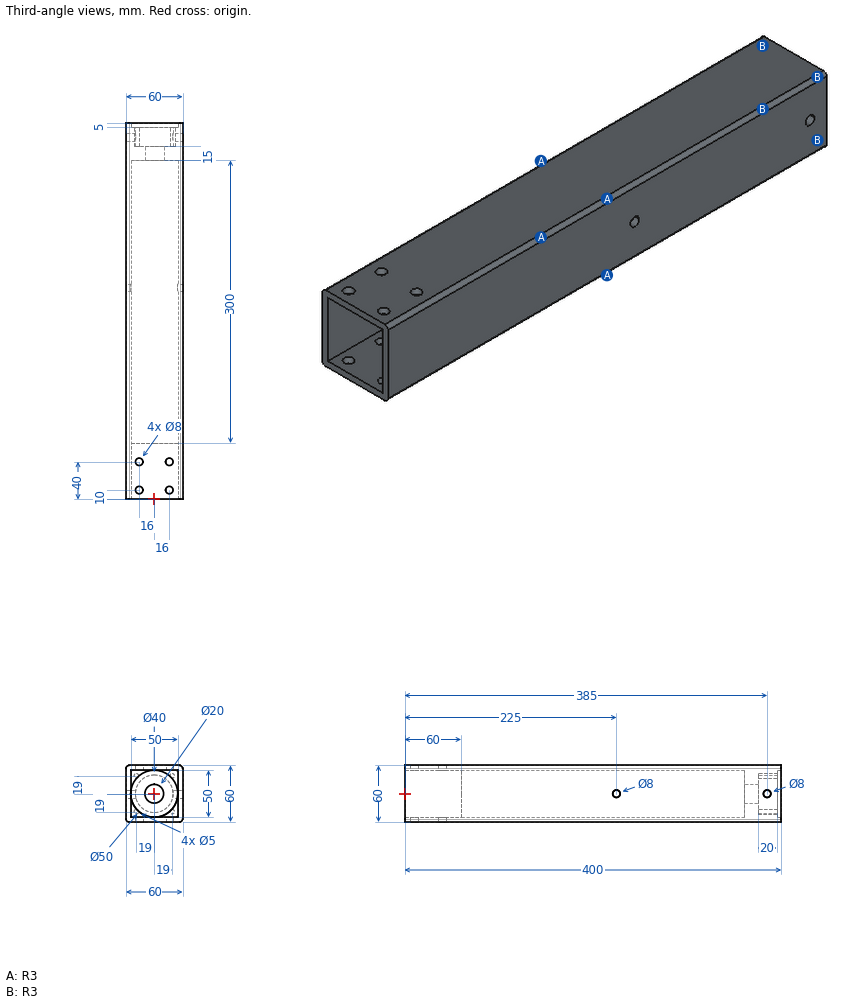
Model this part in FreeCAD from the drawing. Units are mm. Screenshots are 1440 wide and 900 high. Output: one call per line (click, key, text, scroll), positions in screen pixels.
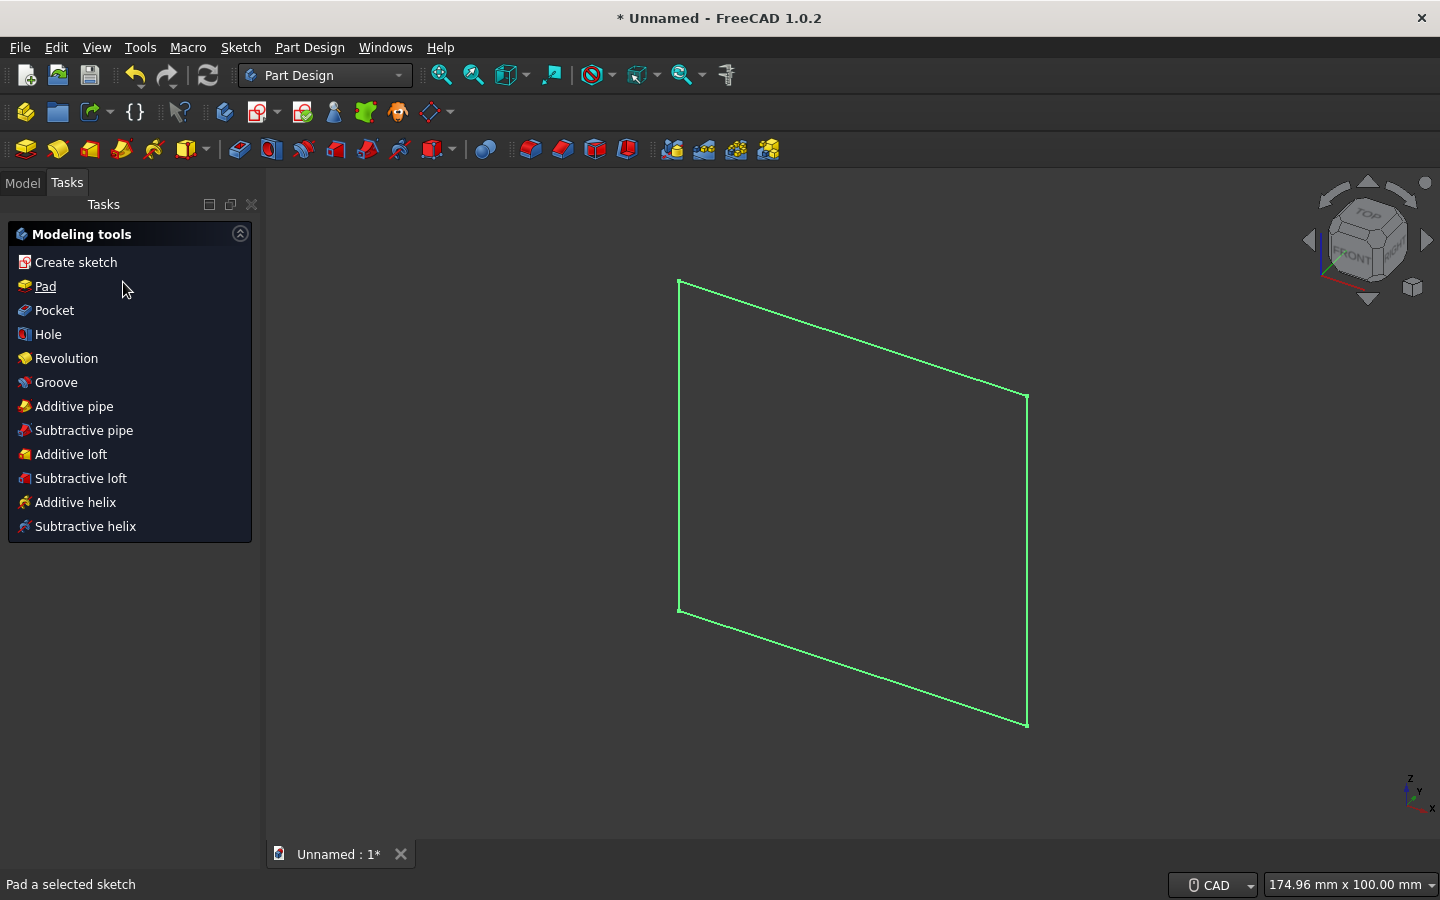
click(26, 150)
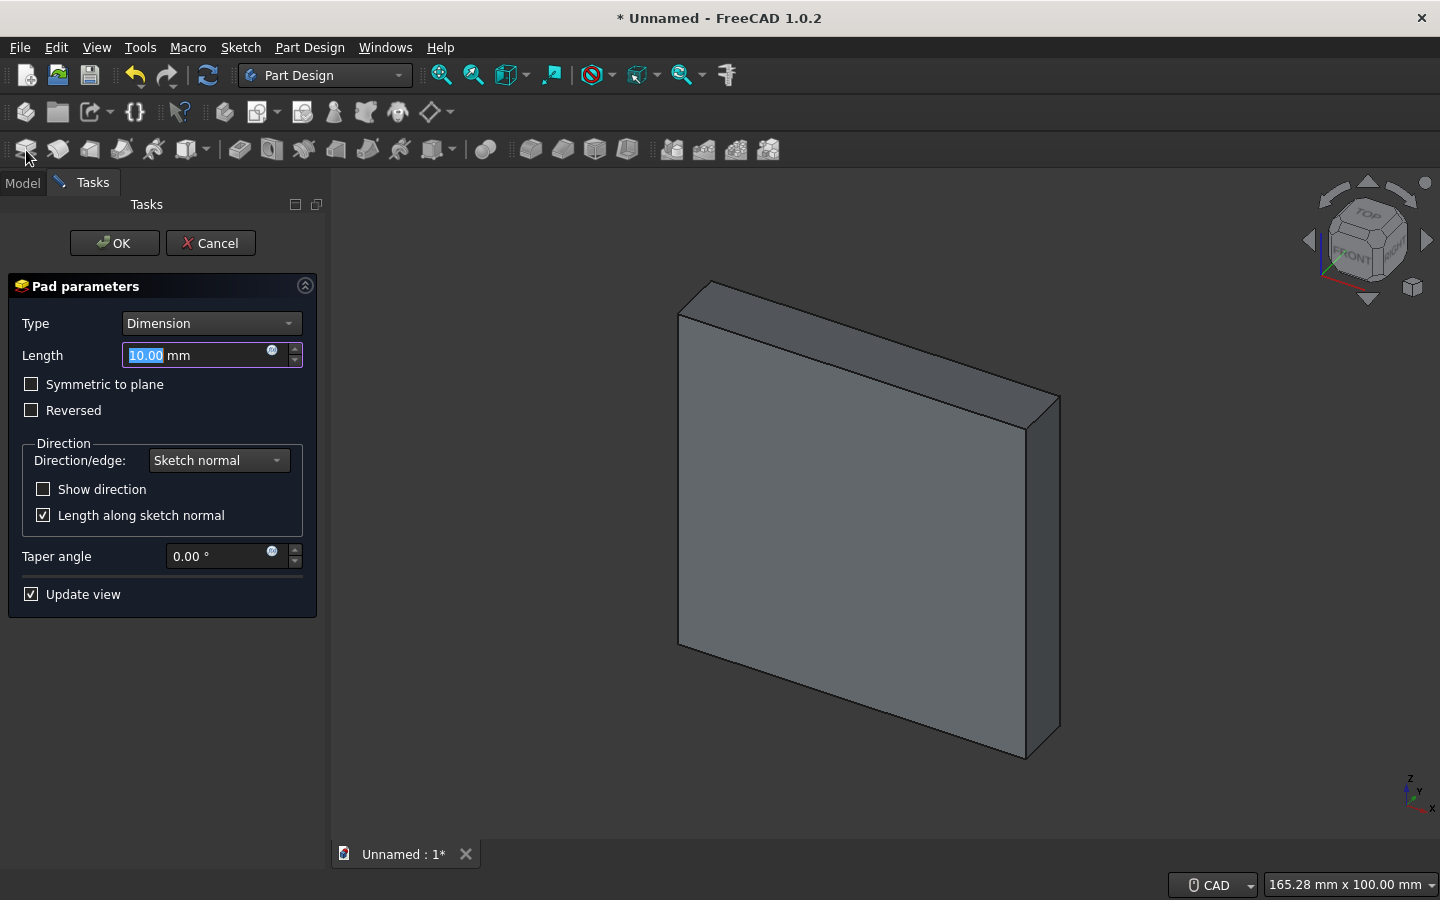
text(400)
key(Tab)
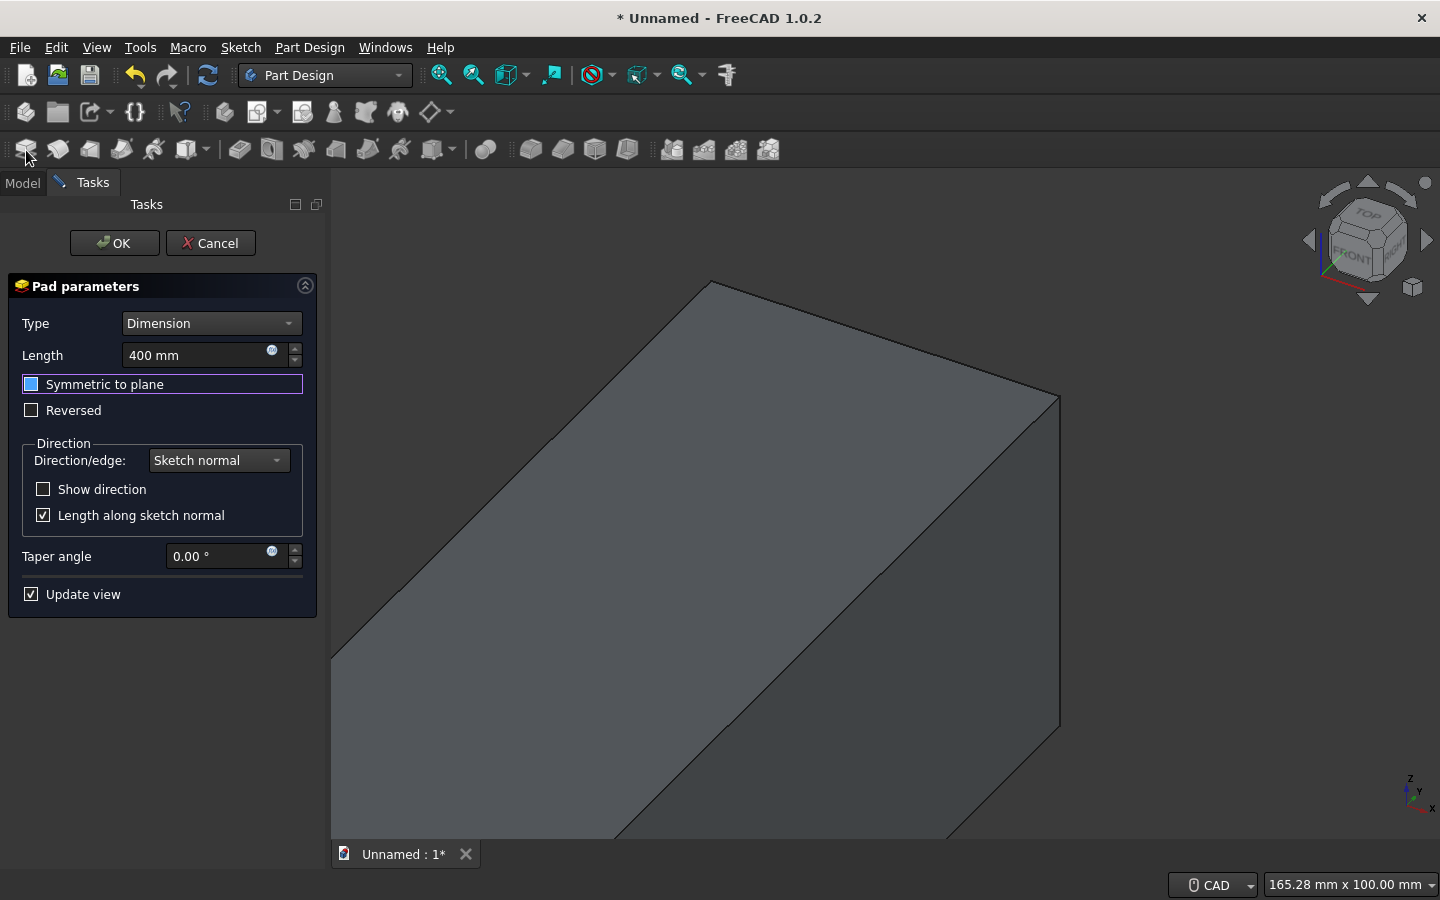
click(30, 410)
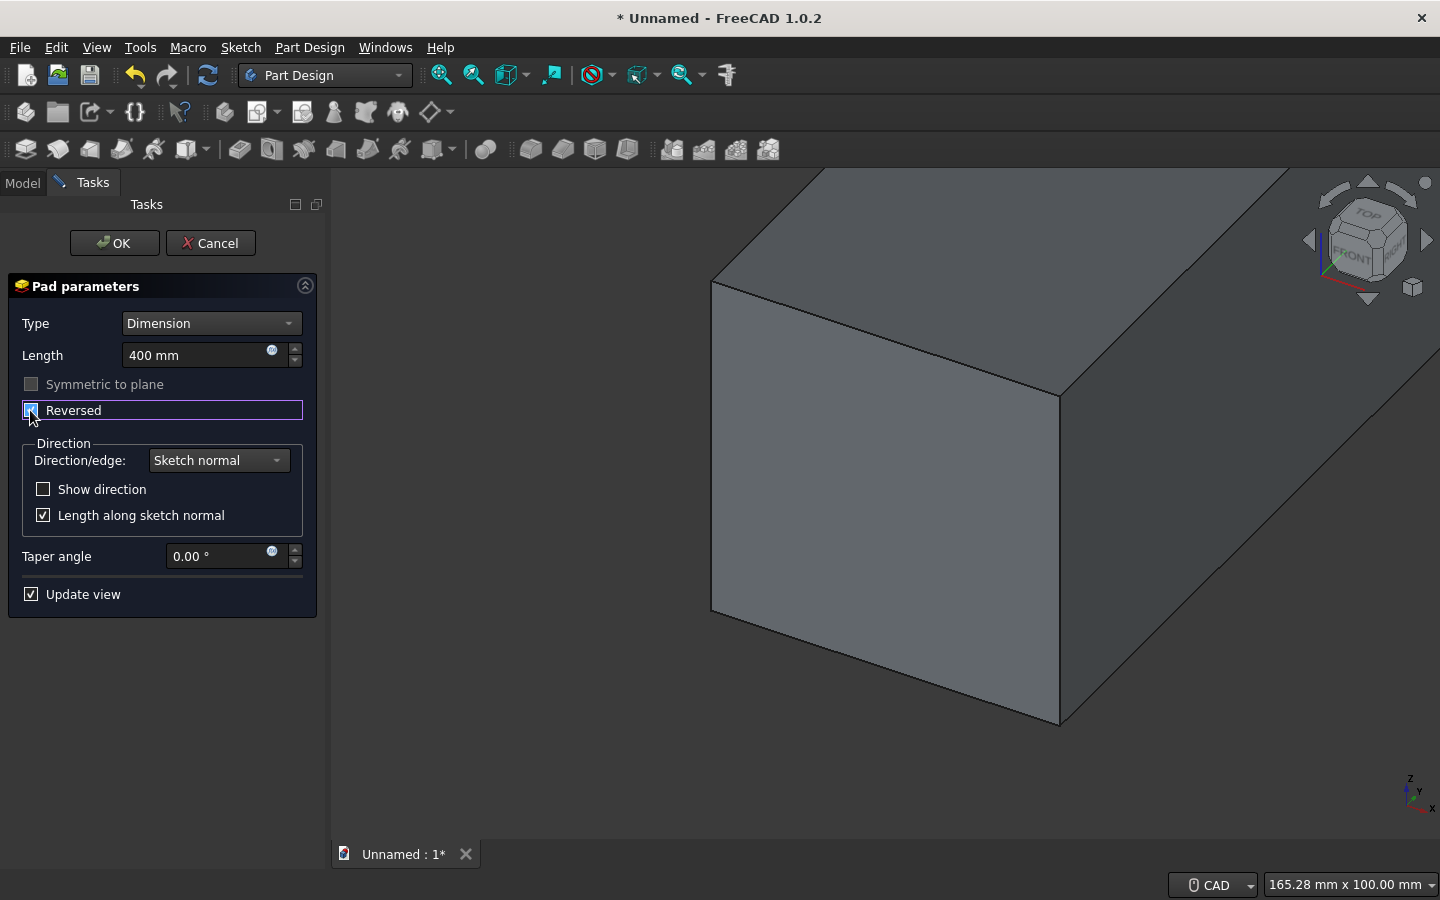
click(115, 243)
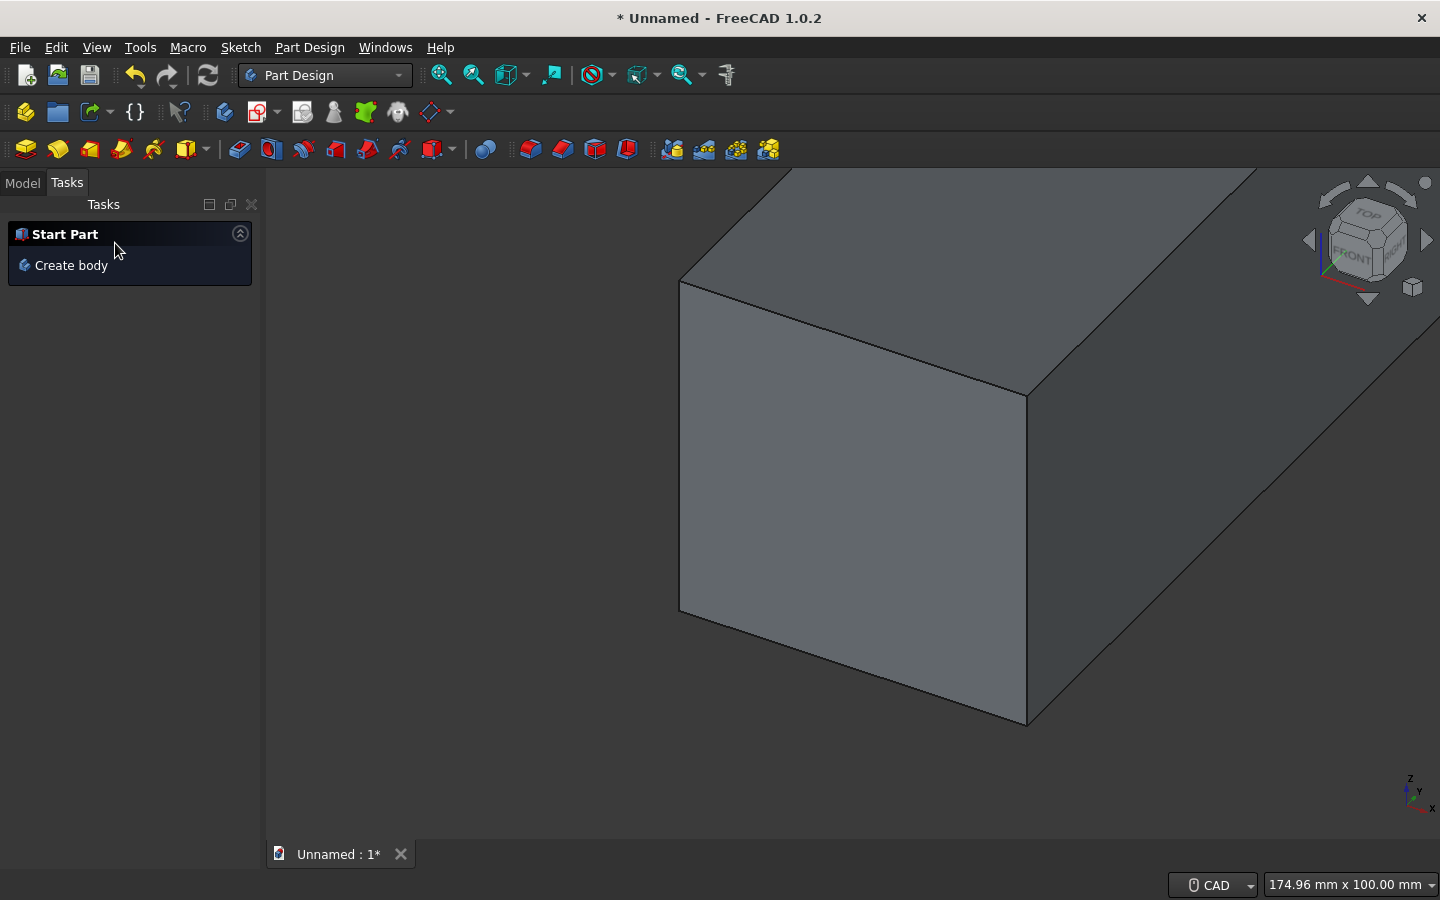
click(442, 76)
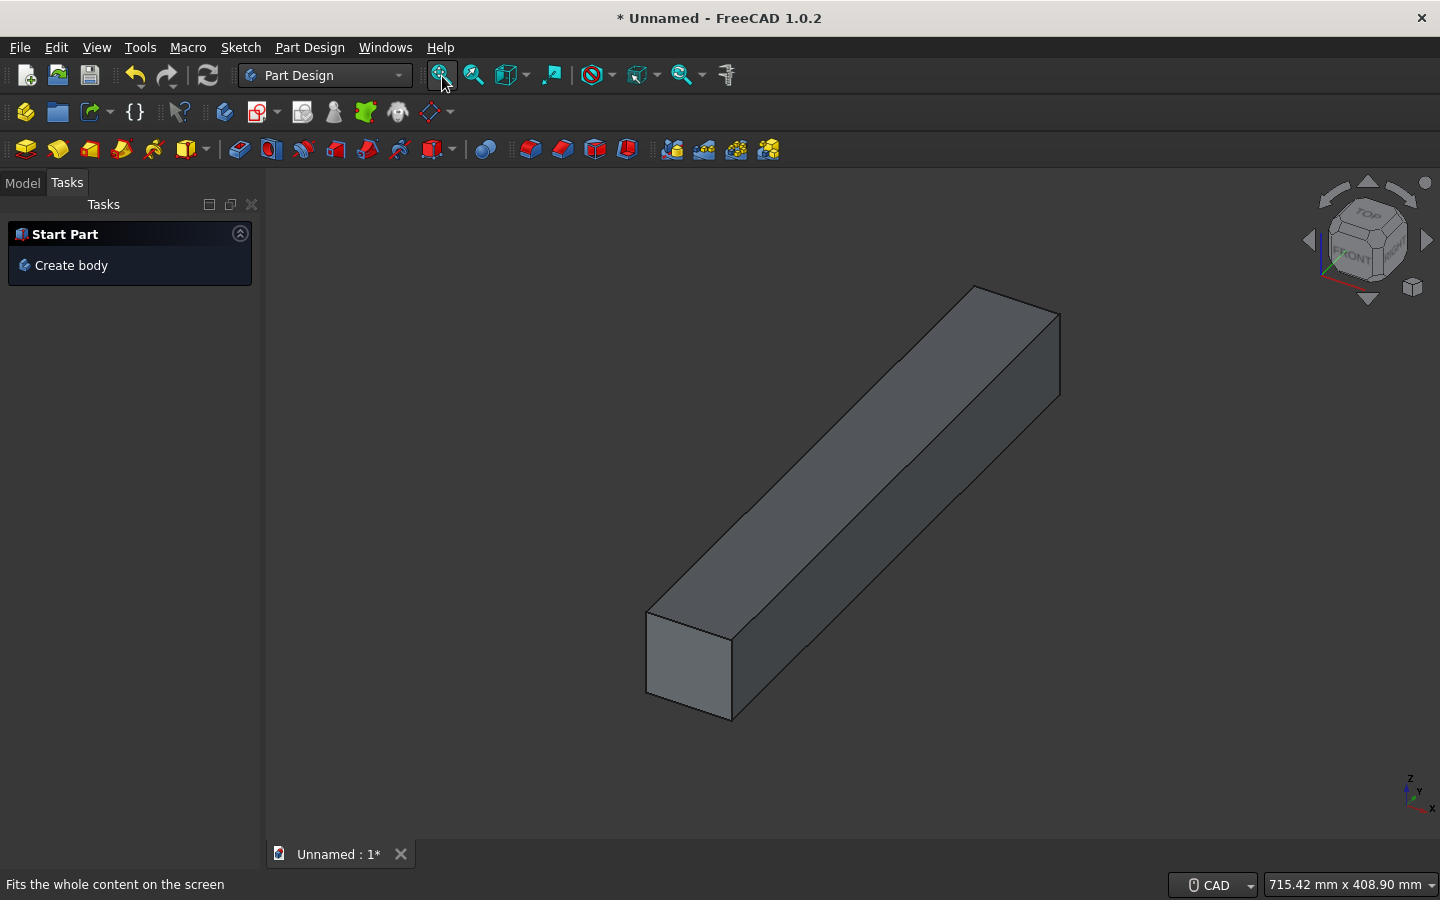
key(4)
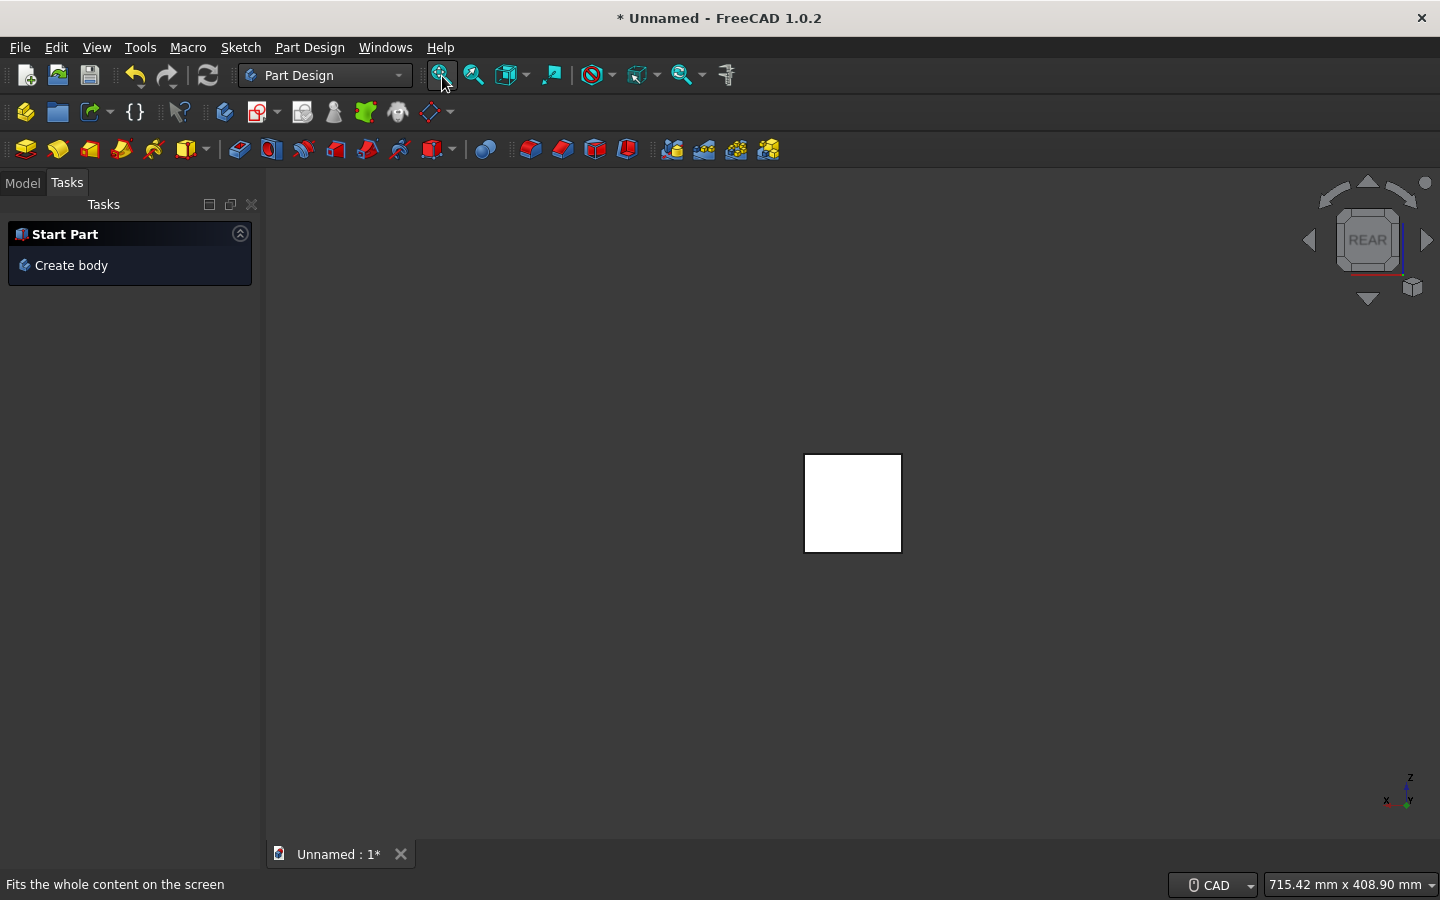
click(442, 76)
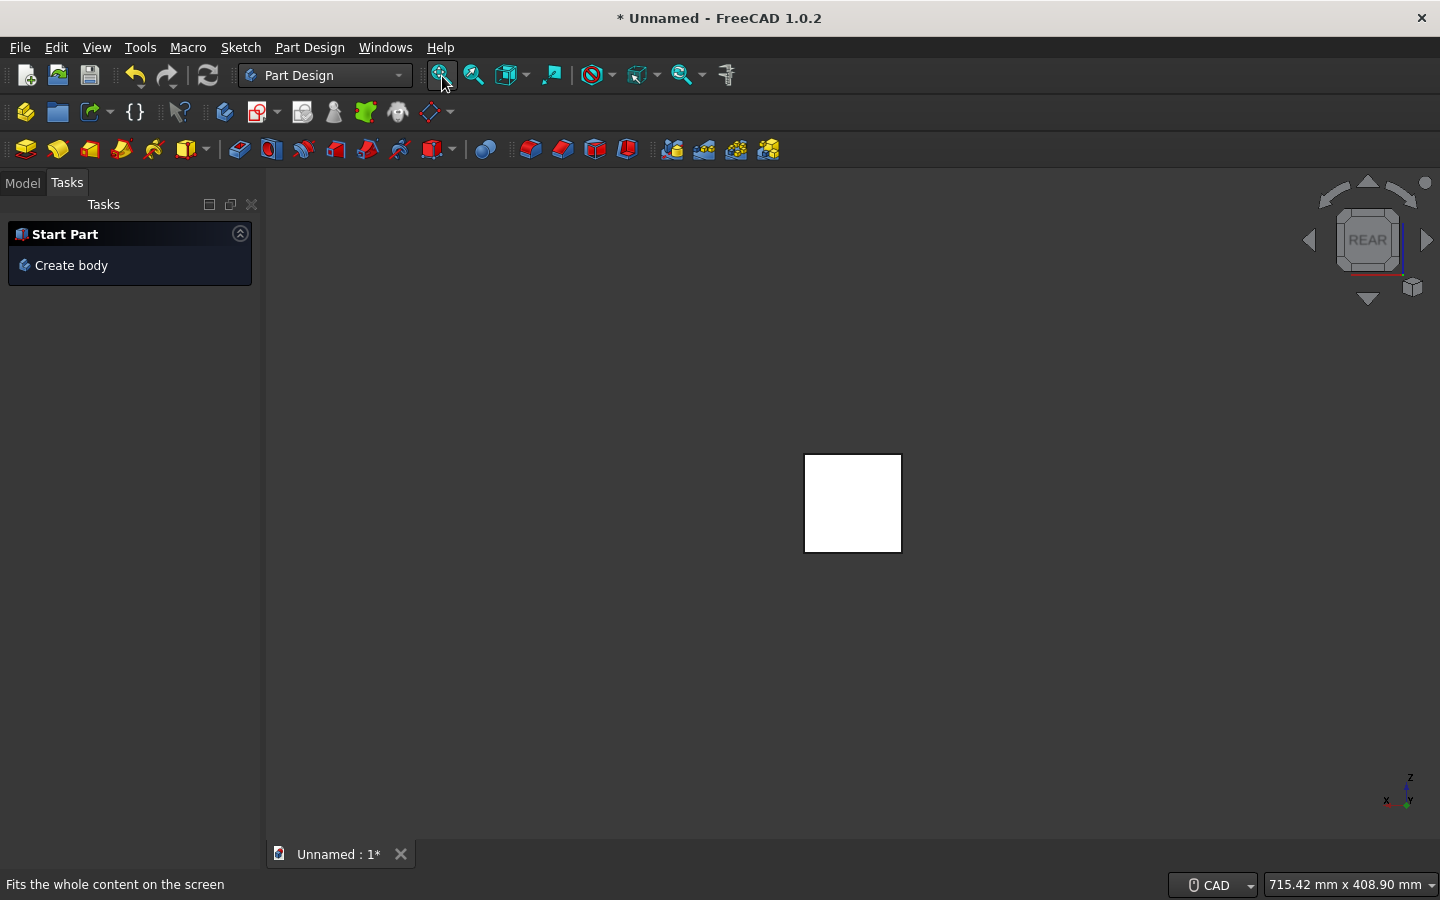
click(853, 503)